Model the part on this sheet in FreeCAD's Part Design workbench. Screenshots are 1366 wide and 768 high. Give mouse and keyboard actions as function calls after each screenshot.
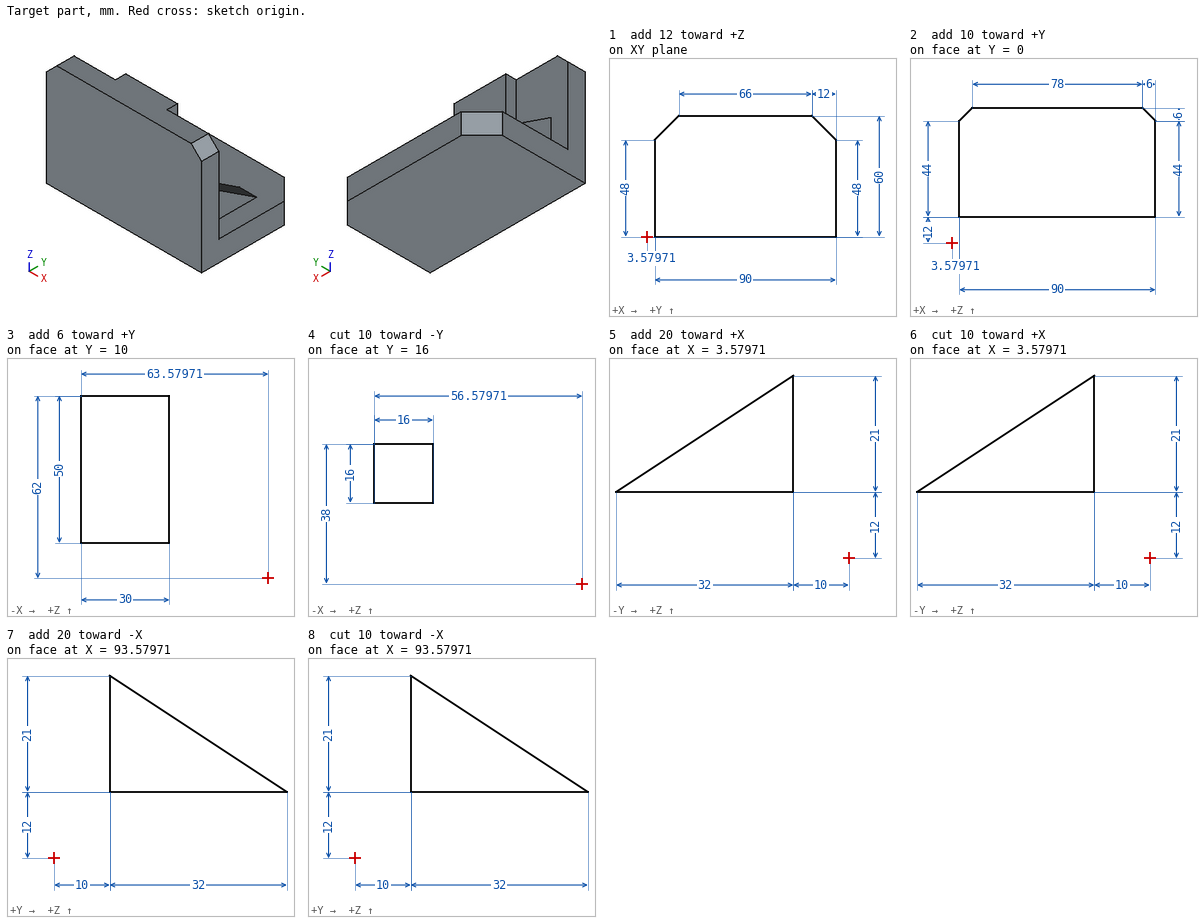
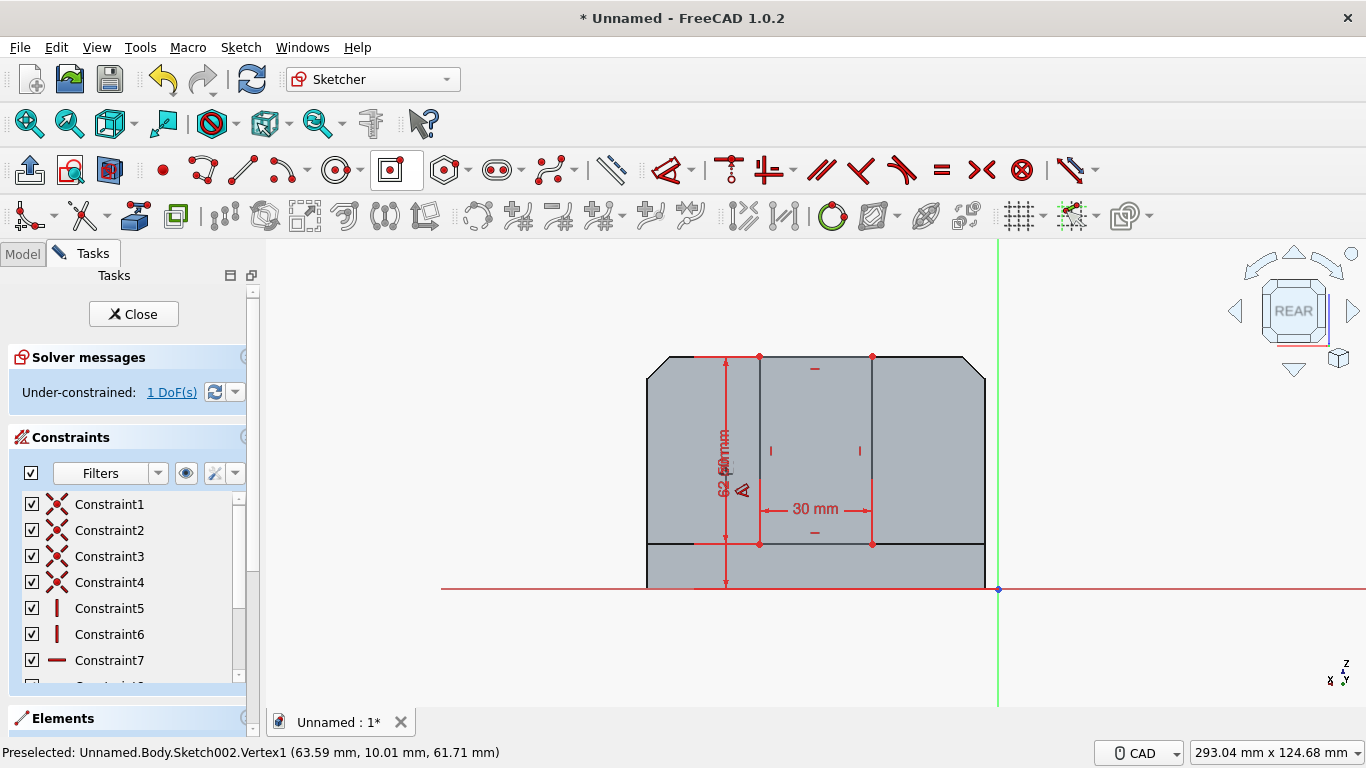
click(760, 357)
click(879, 623)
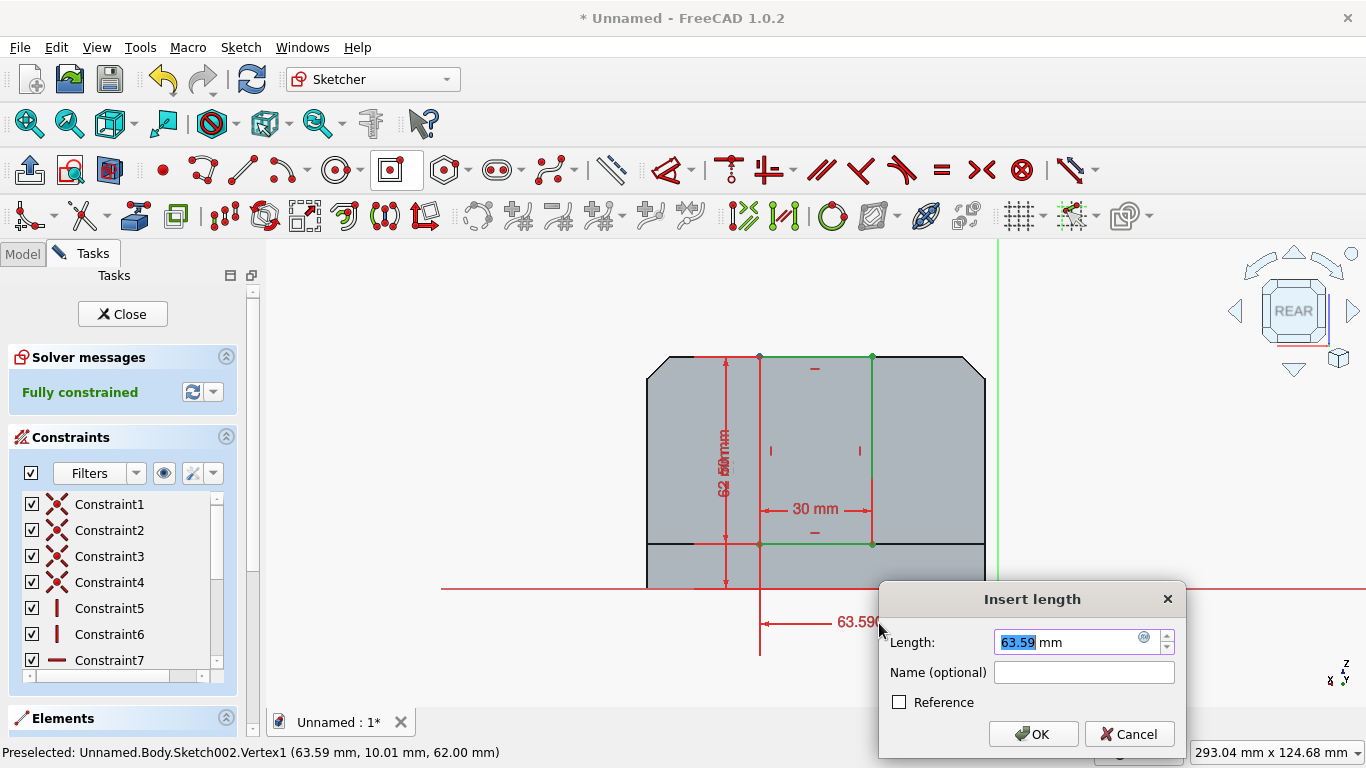
text(63.57971)
key(Return)
key(Escape)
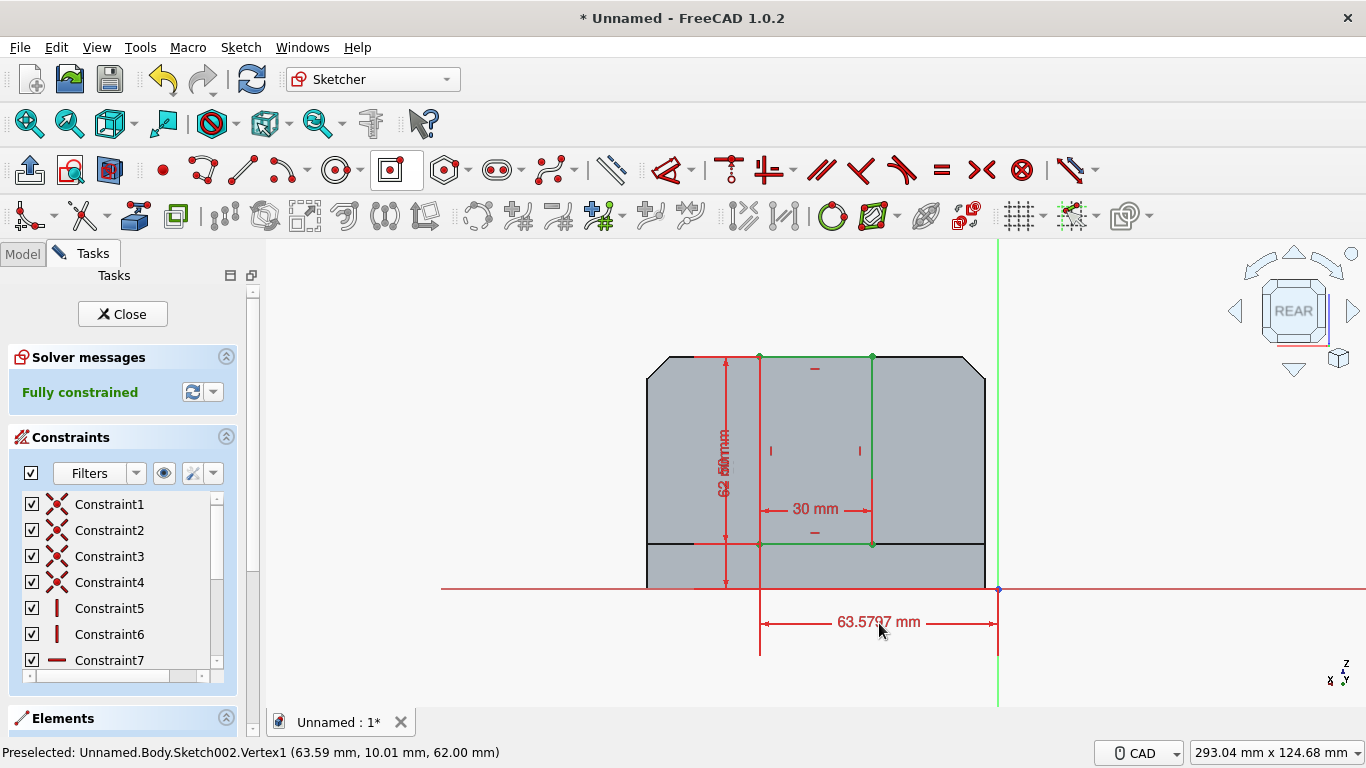
click(123, 314)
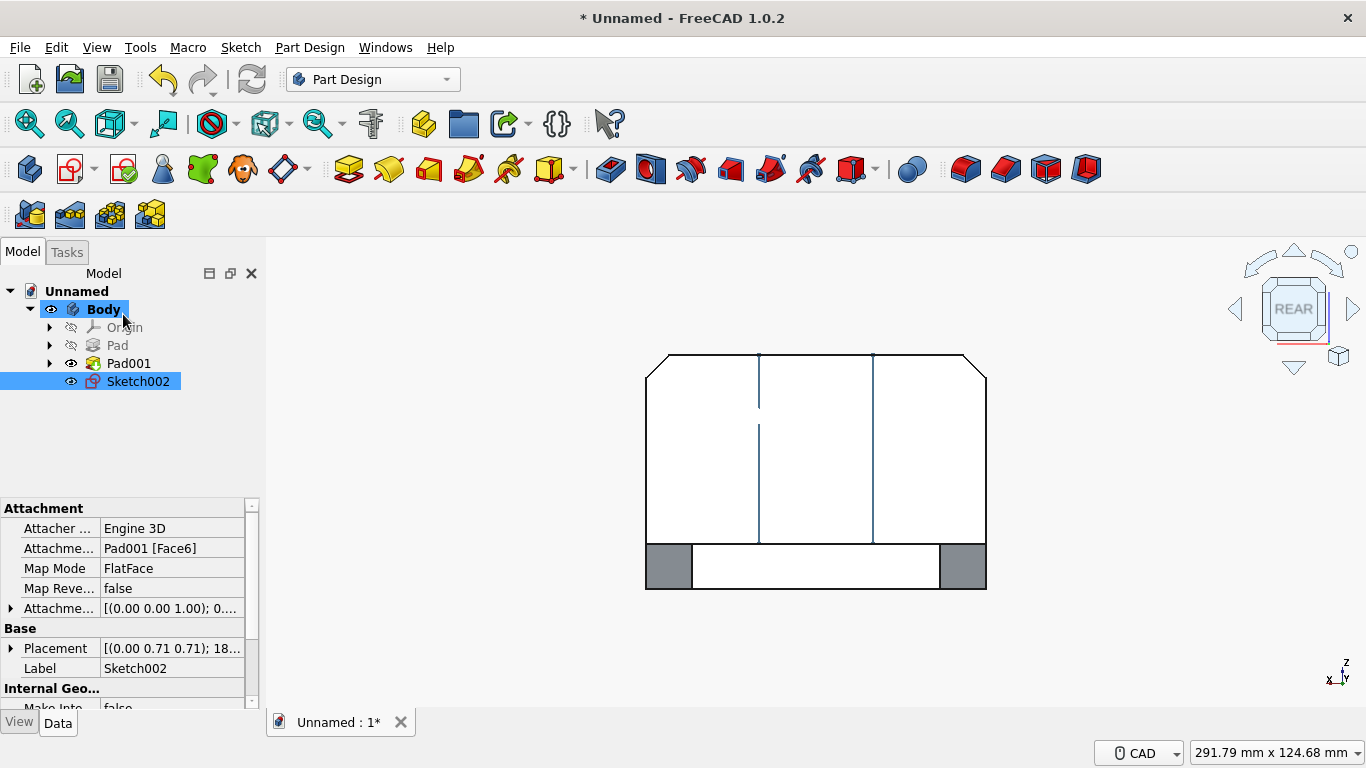
click(350, 170)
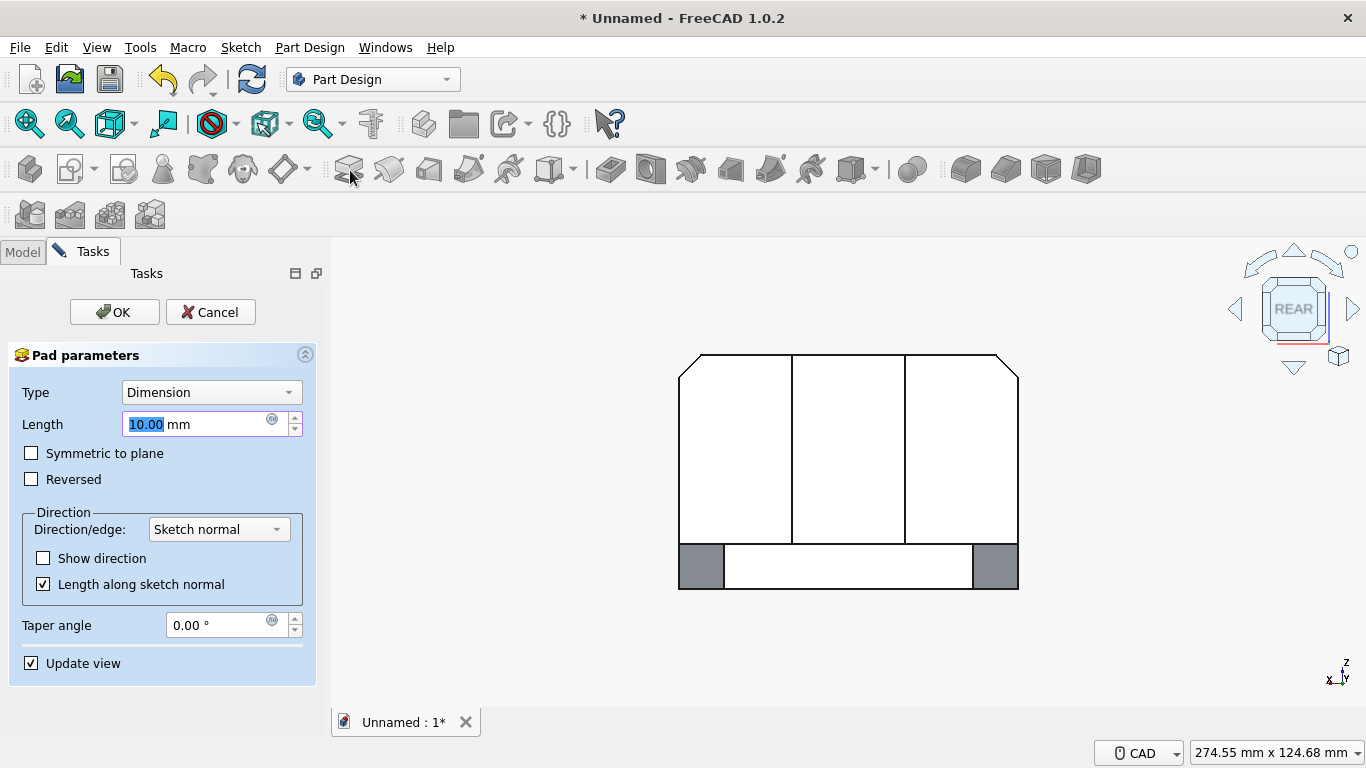
text(6)
key(Tab)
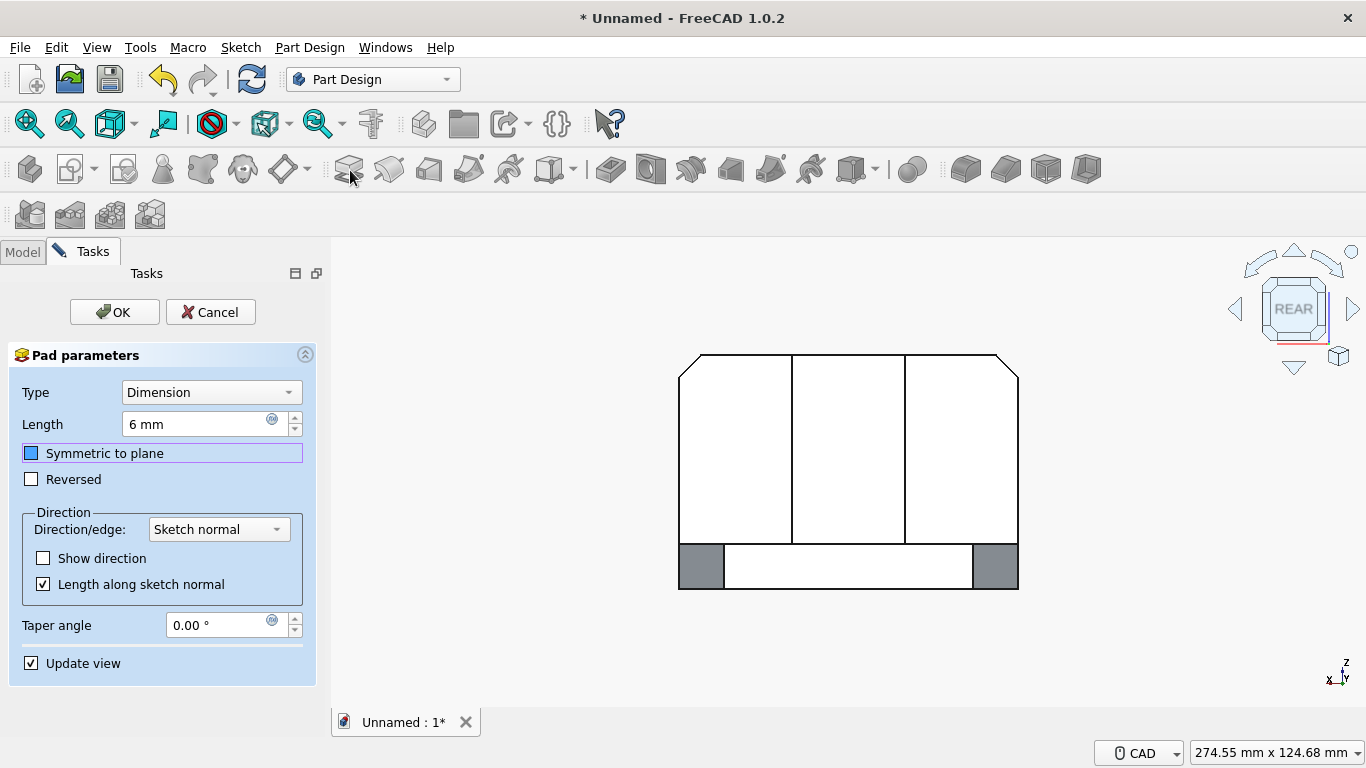
click(115, 312)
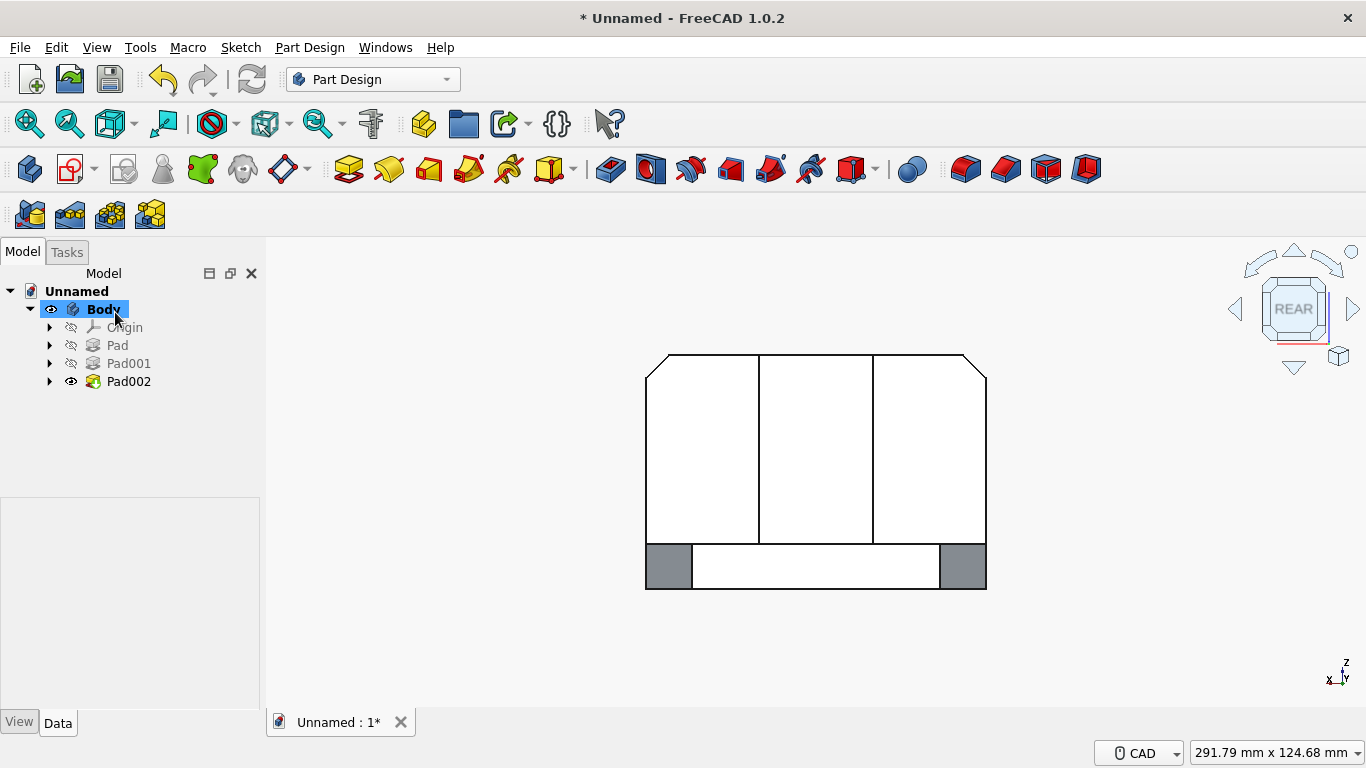
click(816, 421)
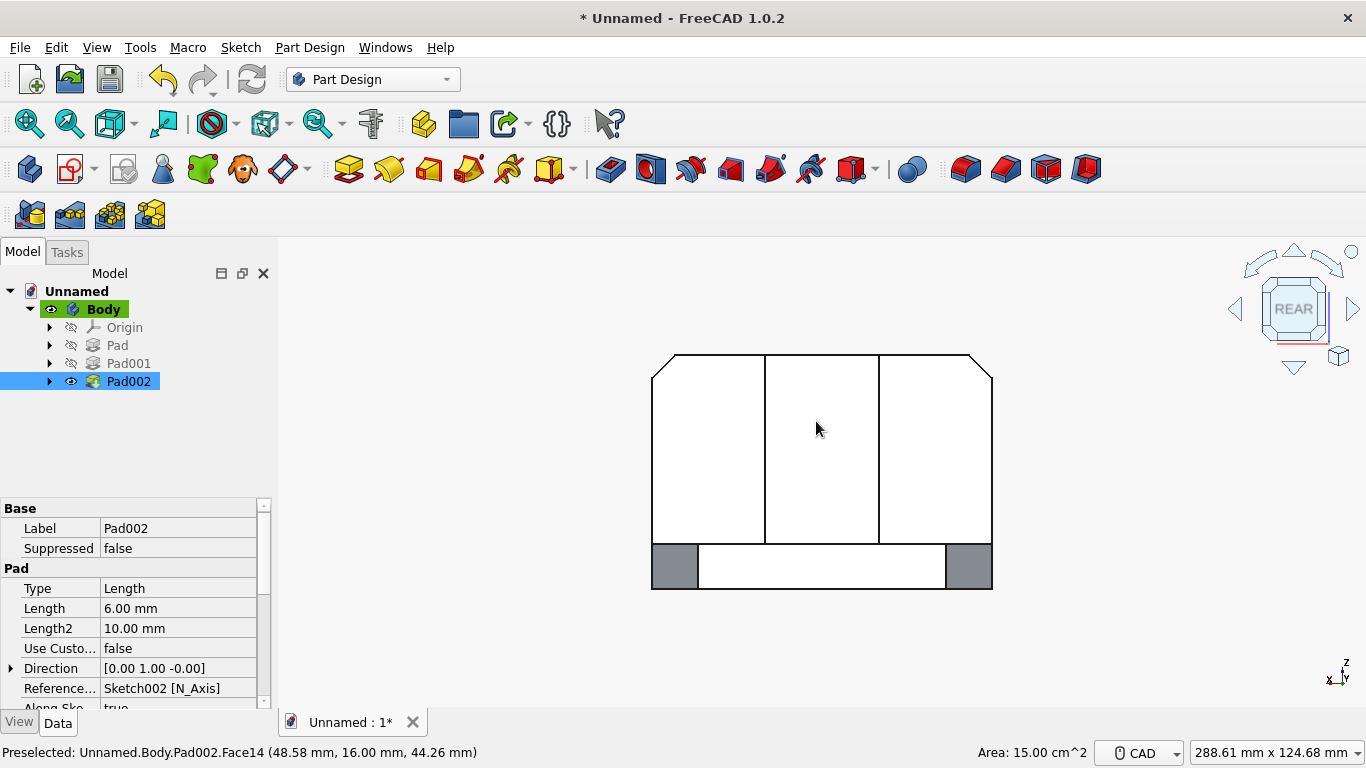
click(70, 170)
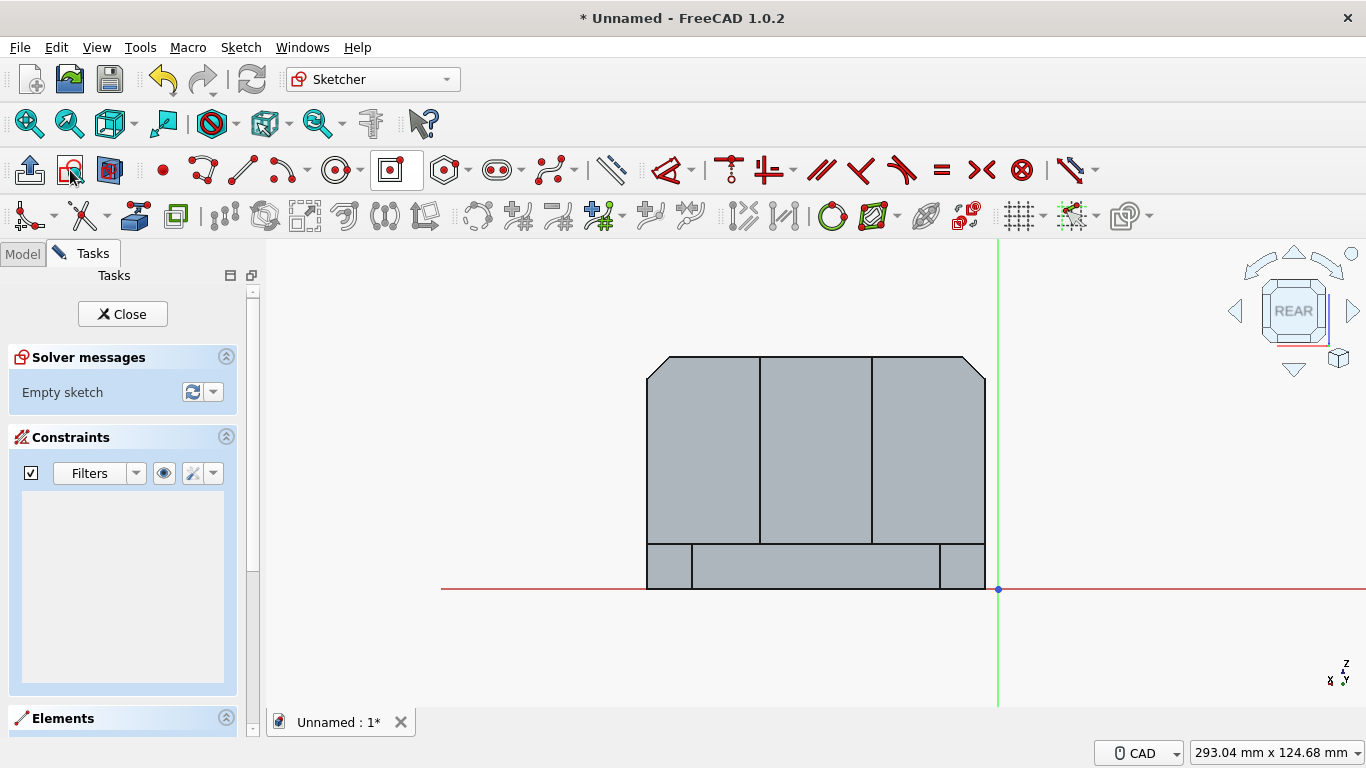
scroll(833, 478, up, 8)